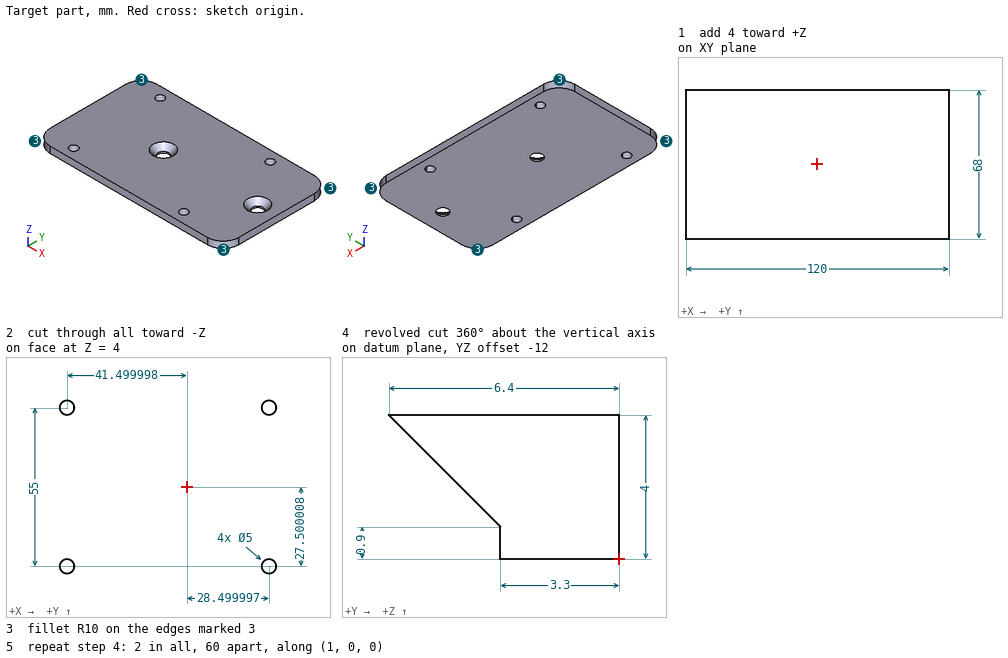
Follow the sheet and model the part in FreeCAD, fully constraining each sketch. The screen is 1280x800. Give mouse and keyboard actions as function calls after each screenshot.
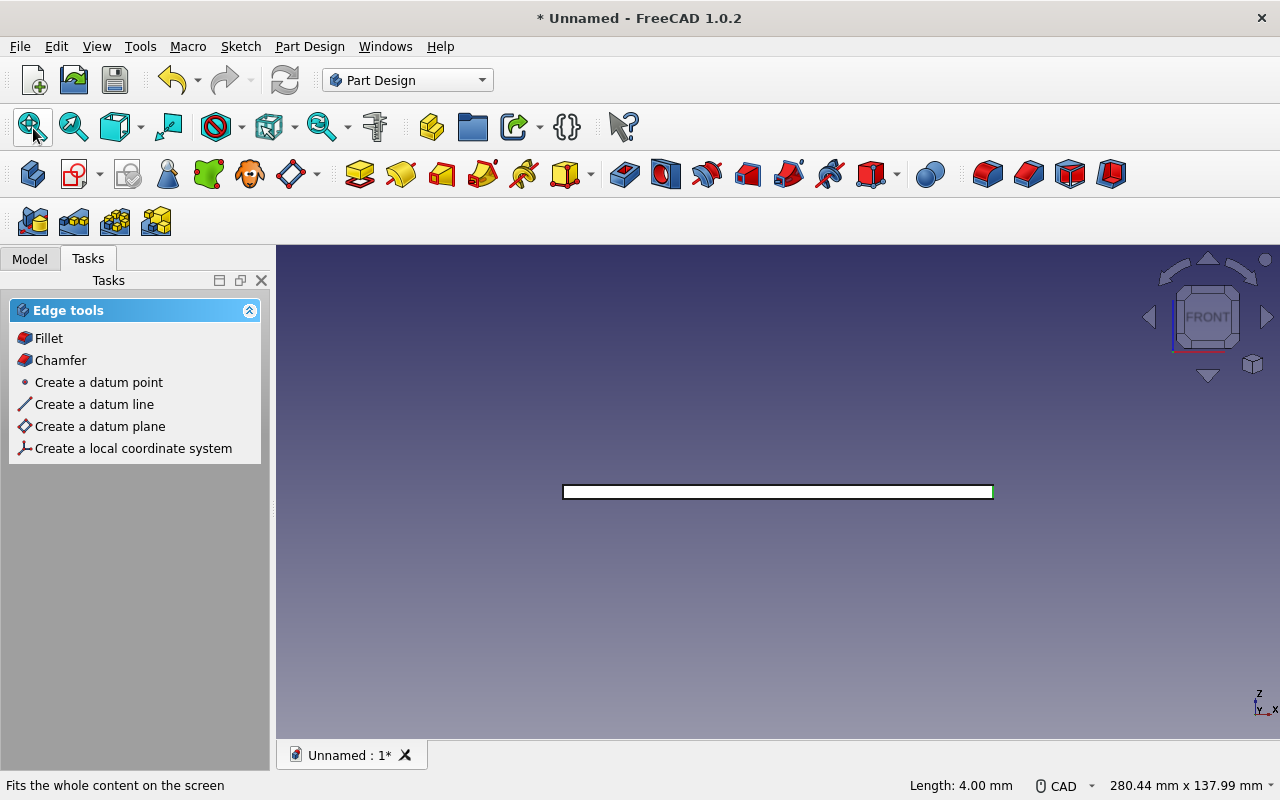
click(33, 128)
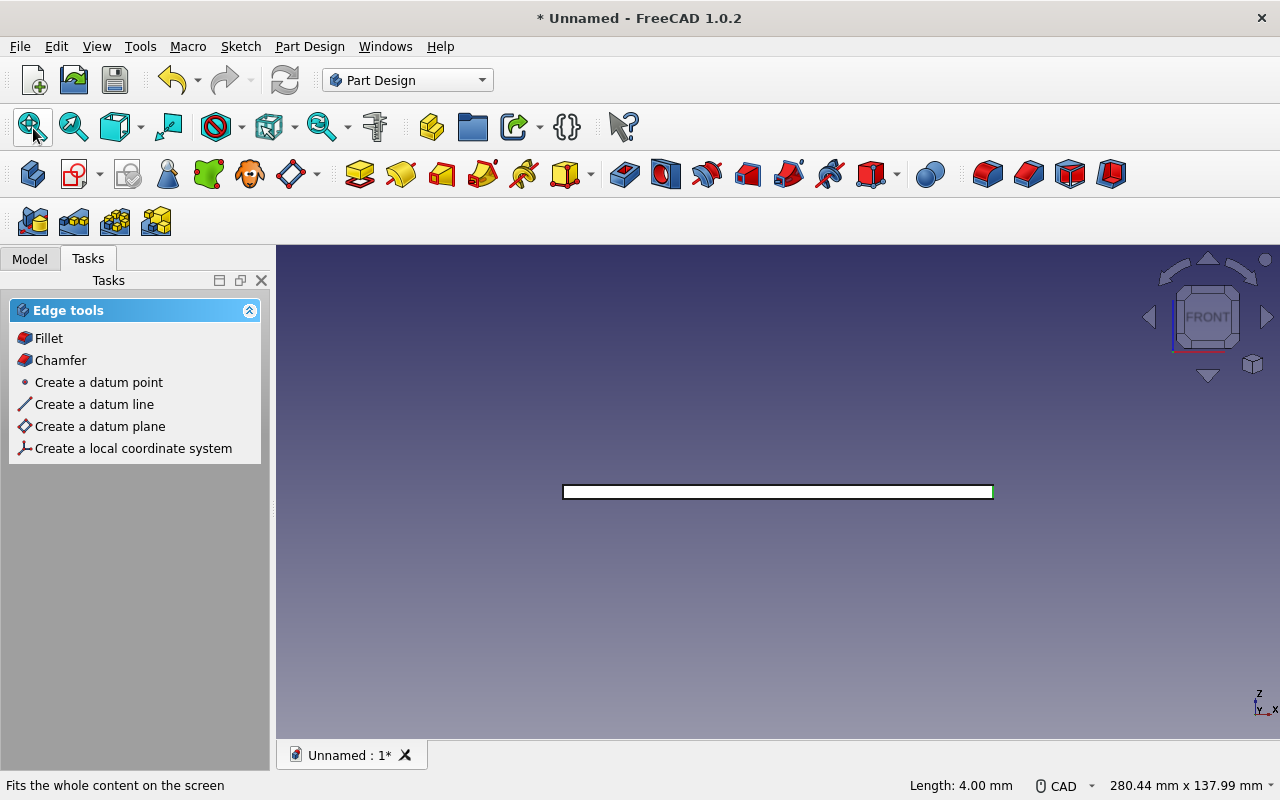
click(563, 491, ctrl)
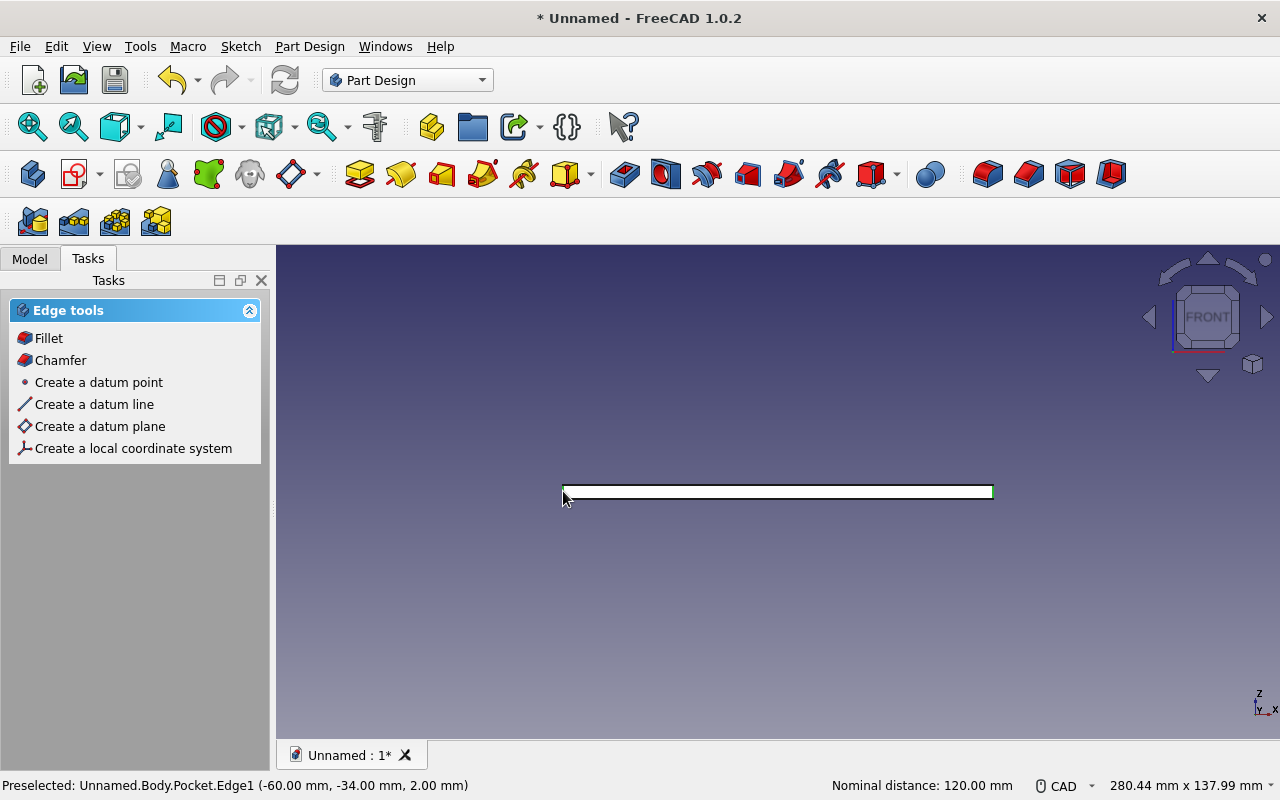
scroll(563, 491, up, 6)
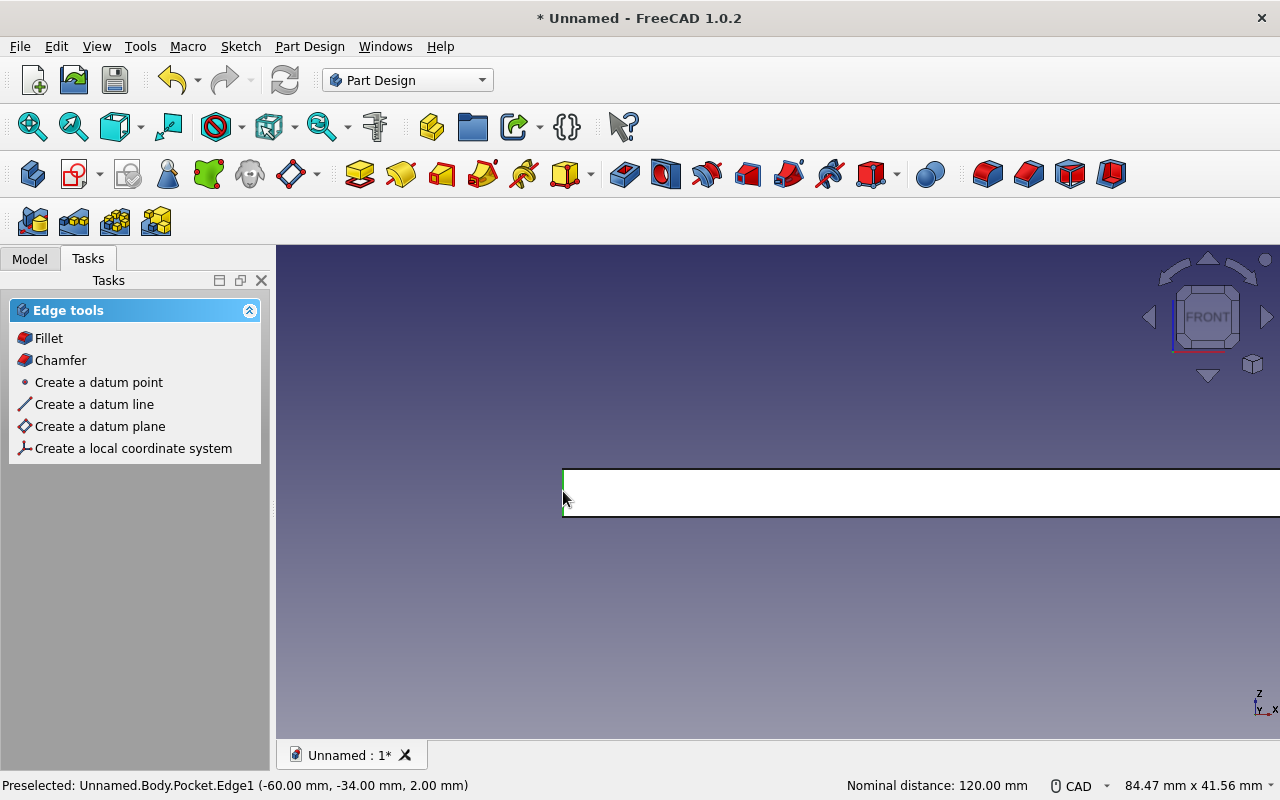
click(33, 128)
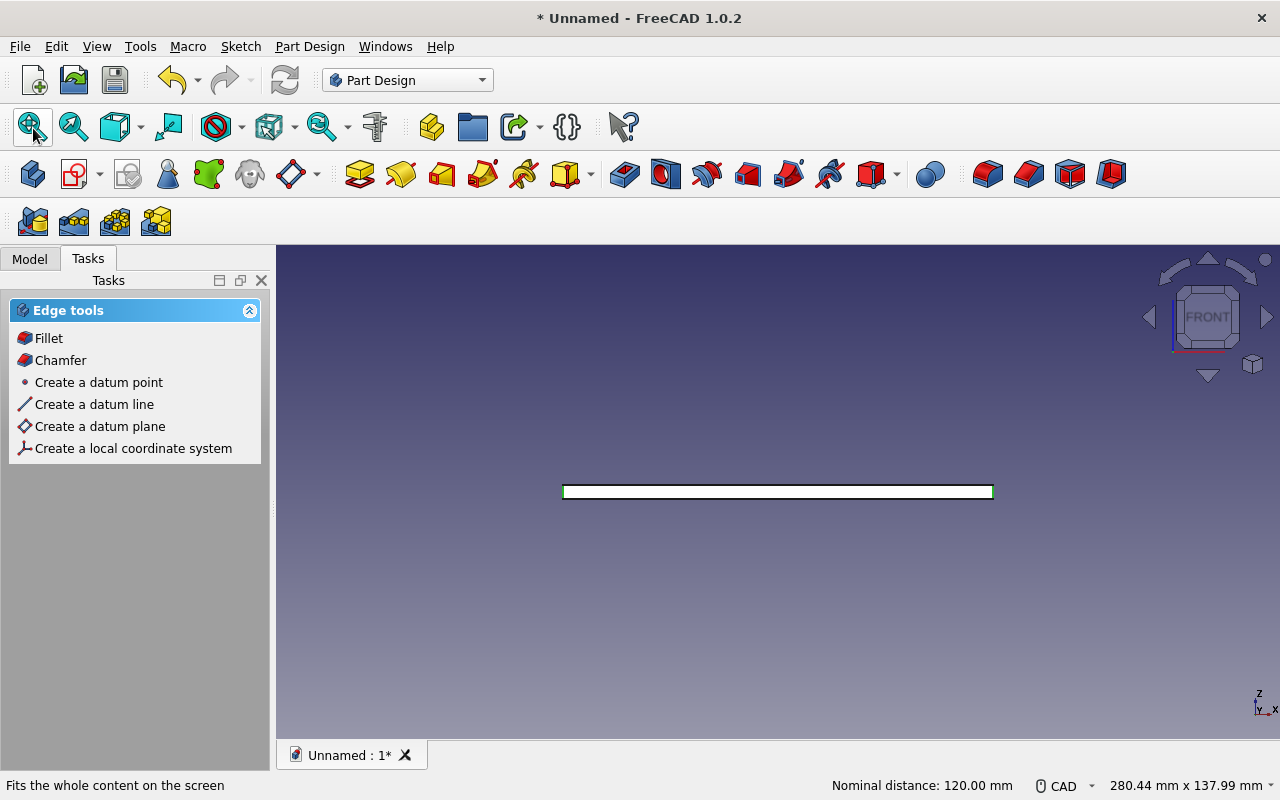
key(3)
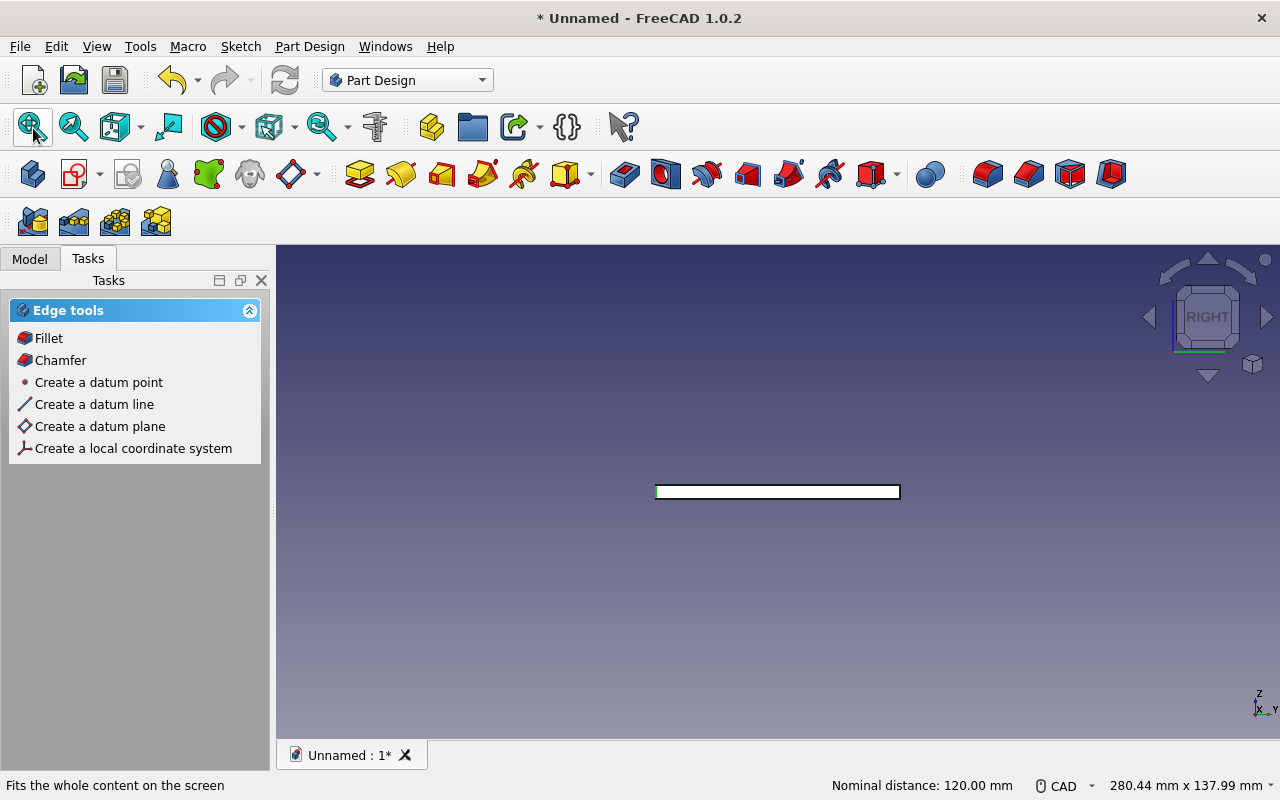
key(v)
key(f)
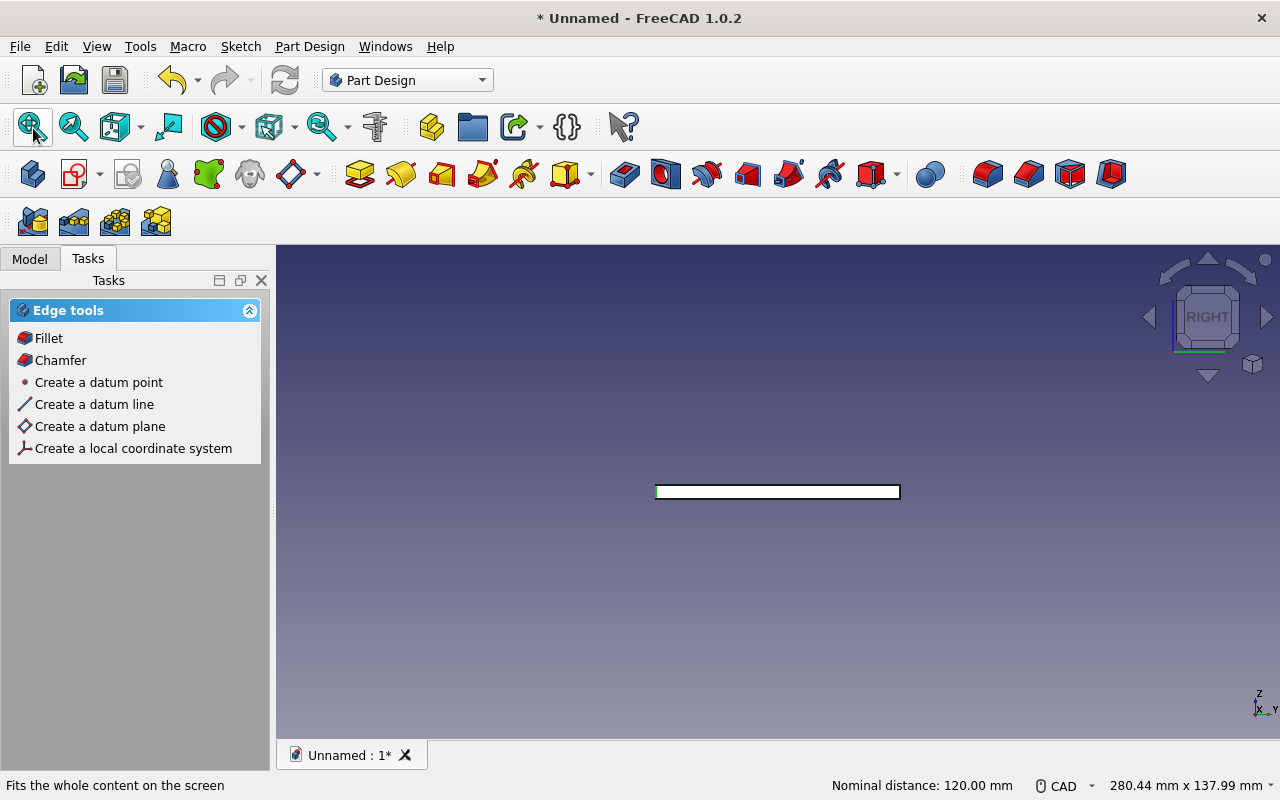
click(900, 491, ctrl)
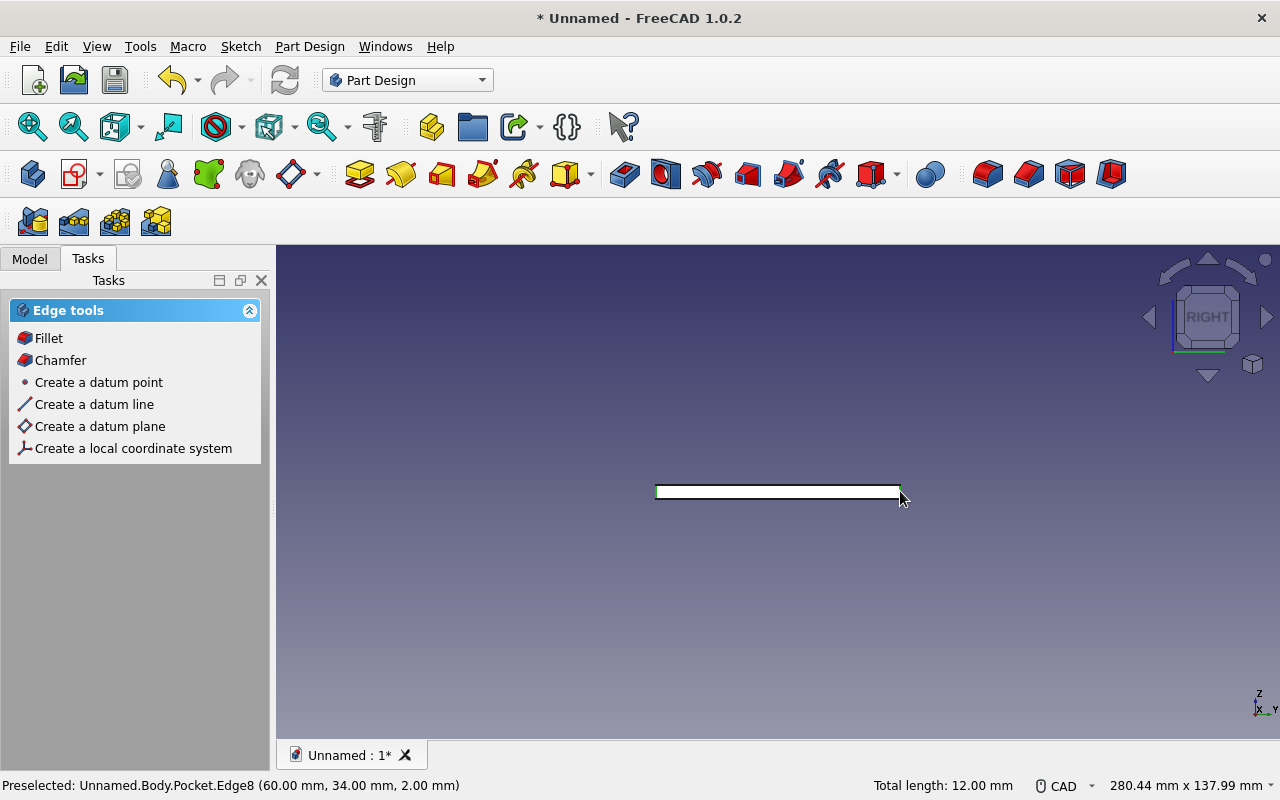
scroll(900, 491, up, 6)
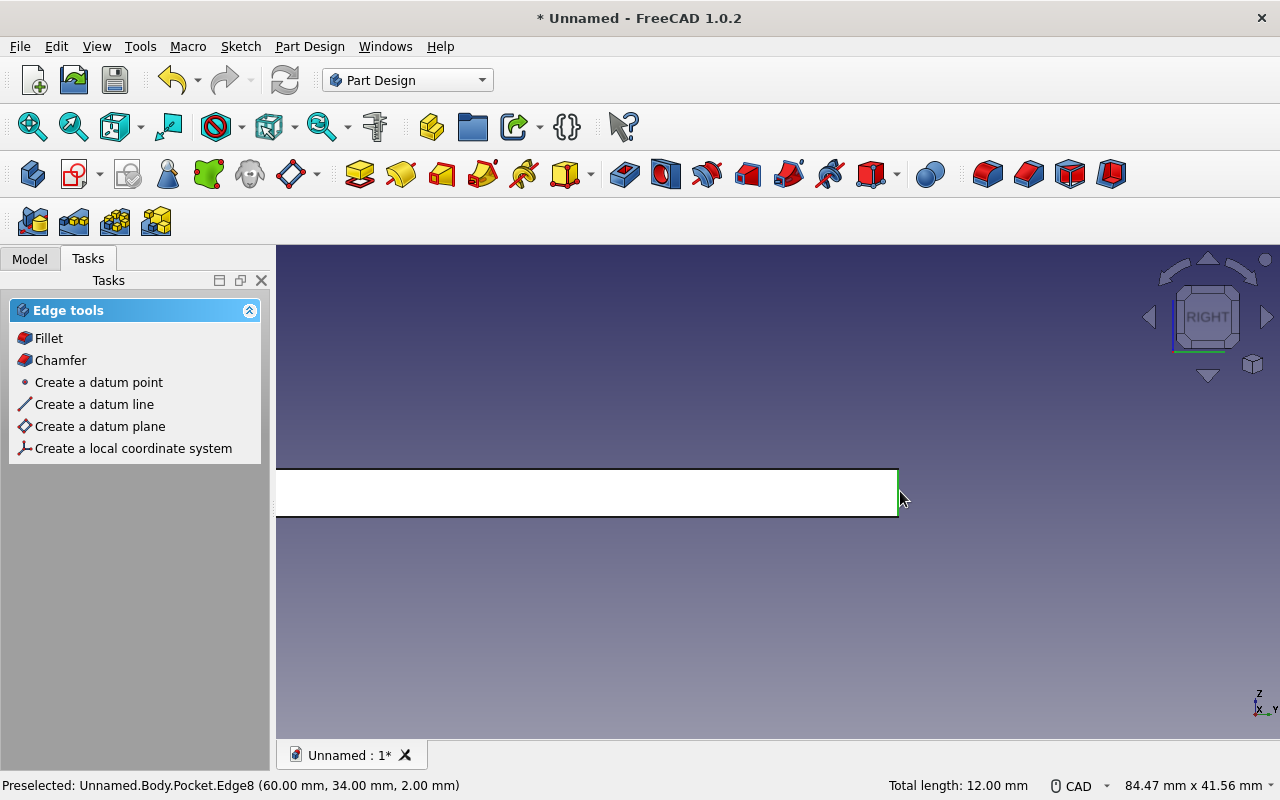
click(33, 128)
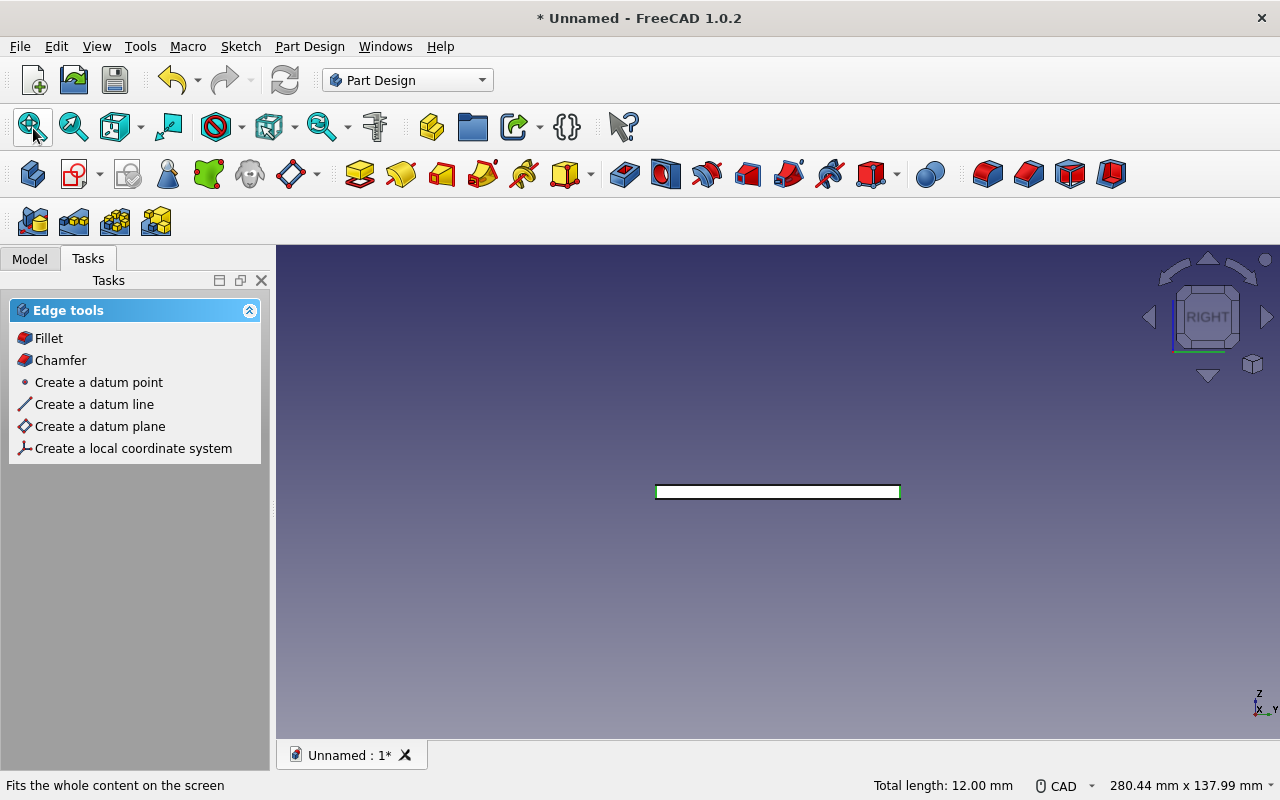
key(5)